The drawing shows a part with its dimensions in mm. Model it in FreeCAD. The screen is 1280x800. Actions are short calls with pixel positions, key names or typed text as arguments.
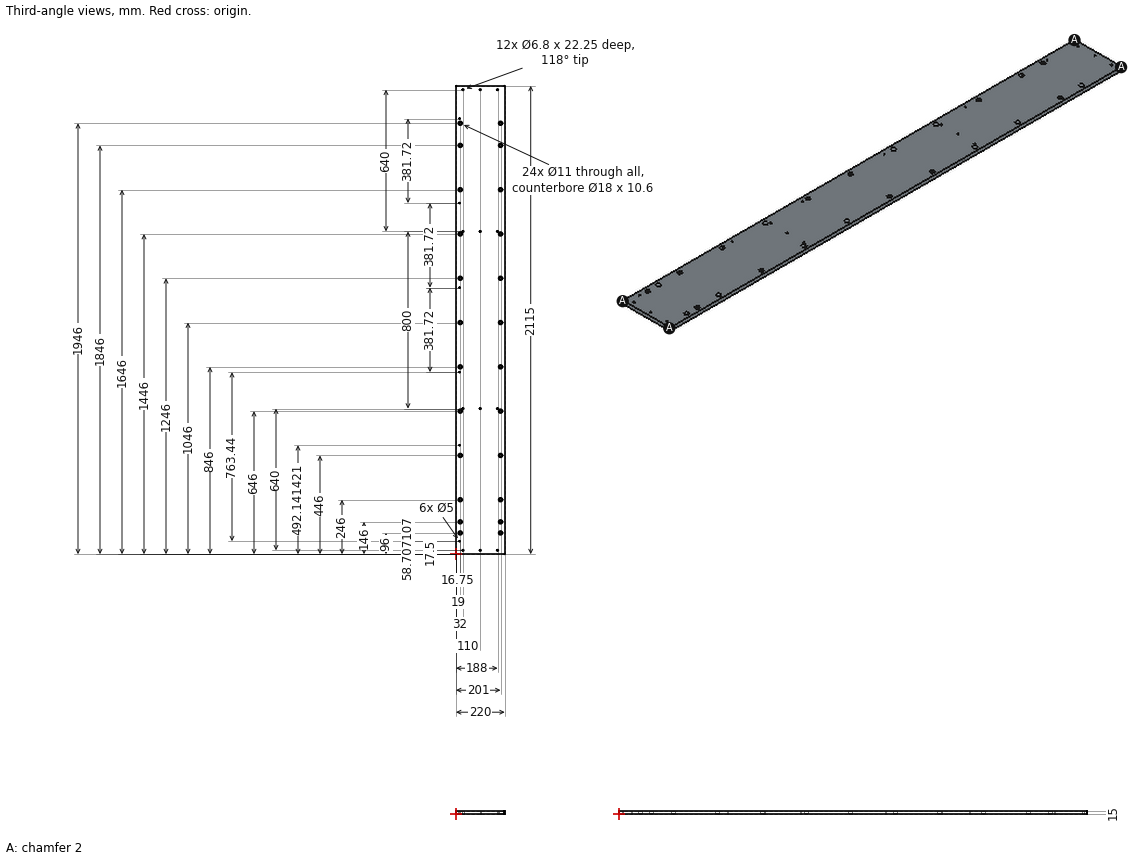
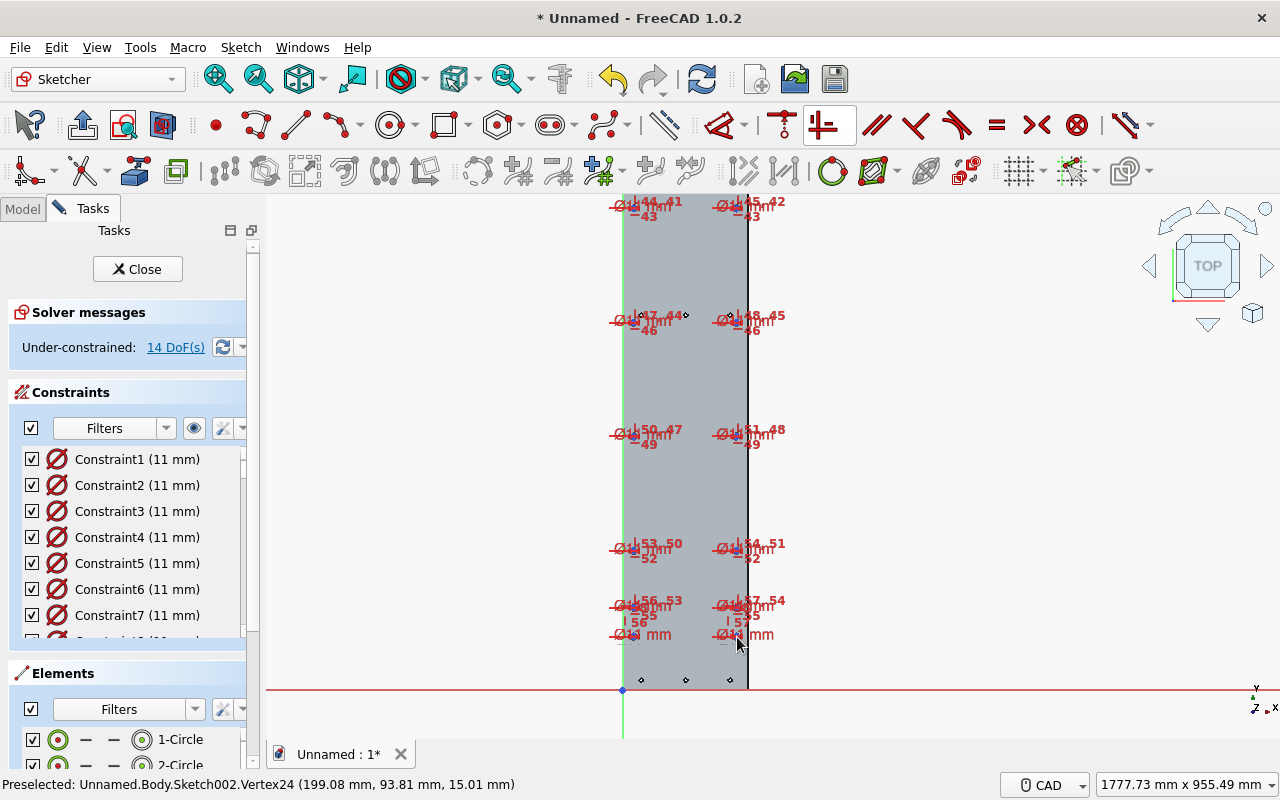
click(720, 126)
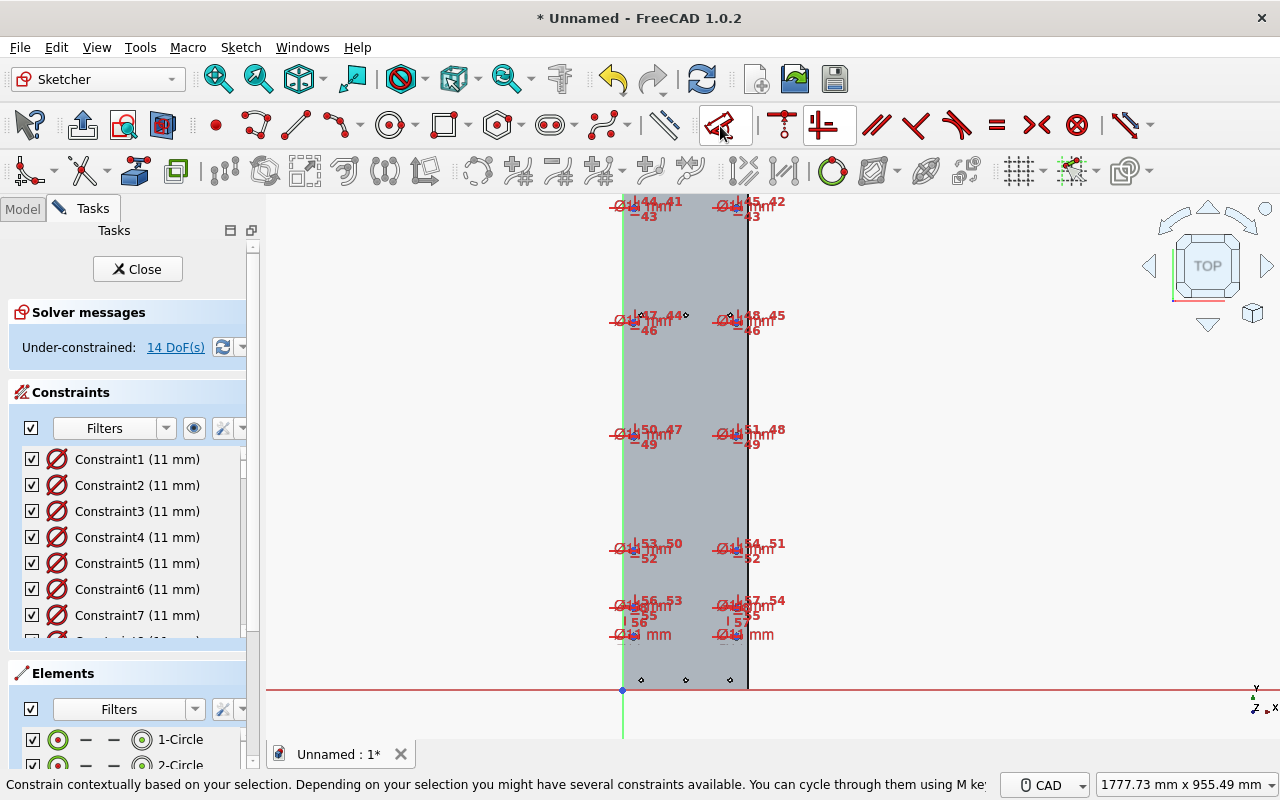
scroll(714, 610, down, 6)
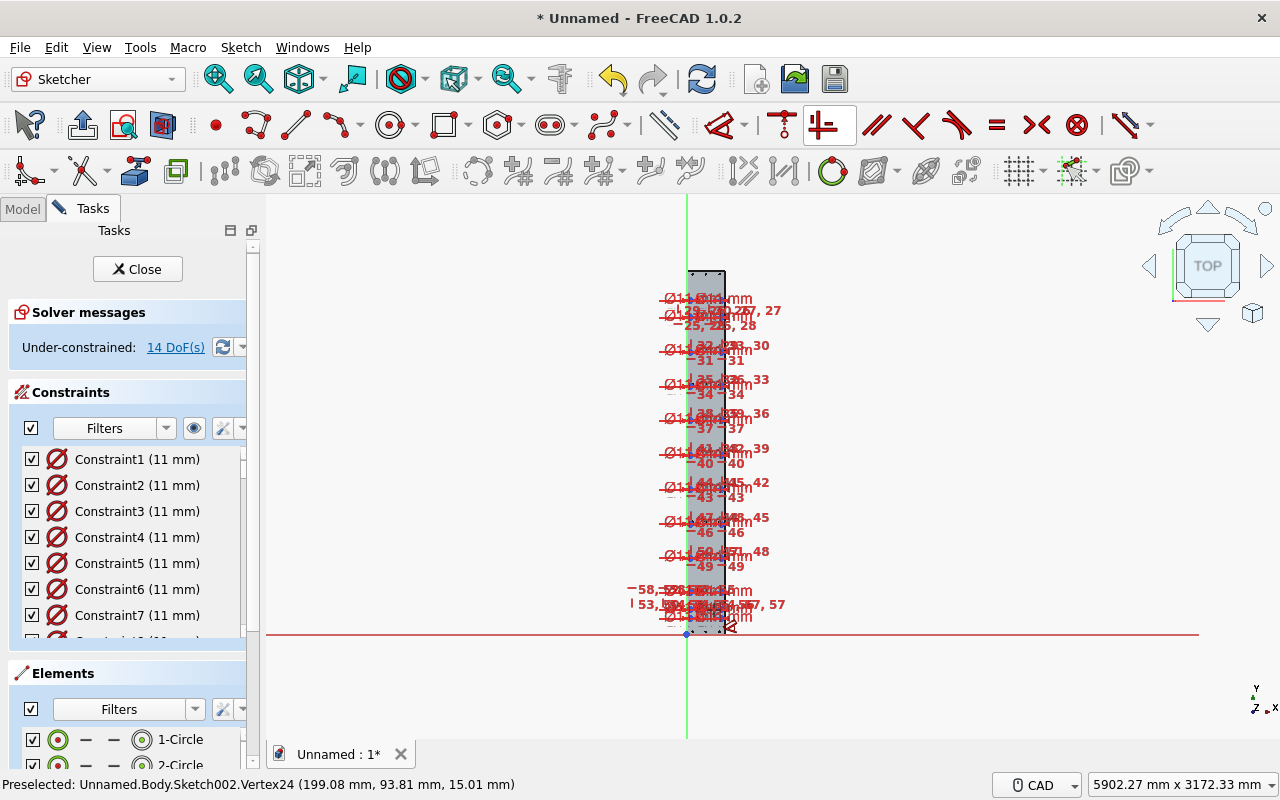
scroll(690, 301, up, 13)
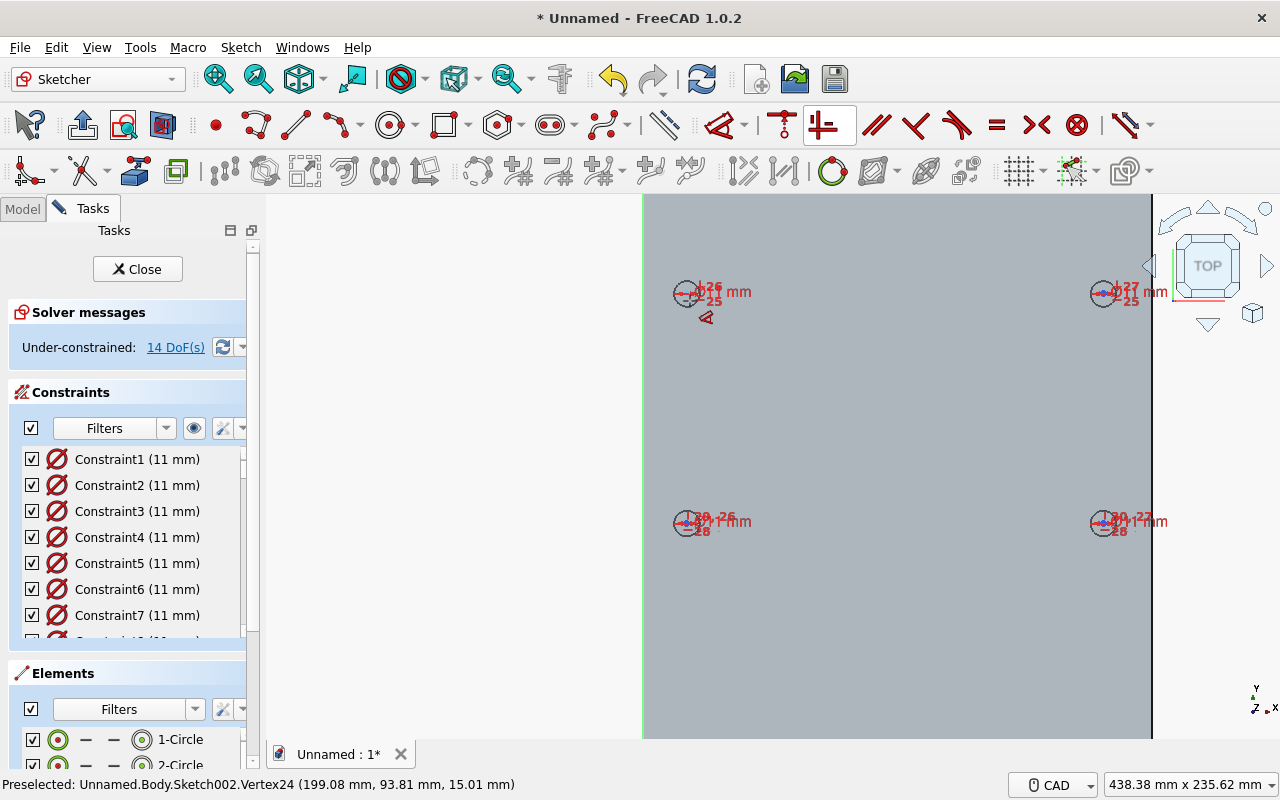
click(687, 294)
click(665, 260)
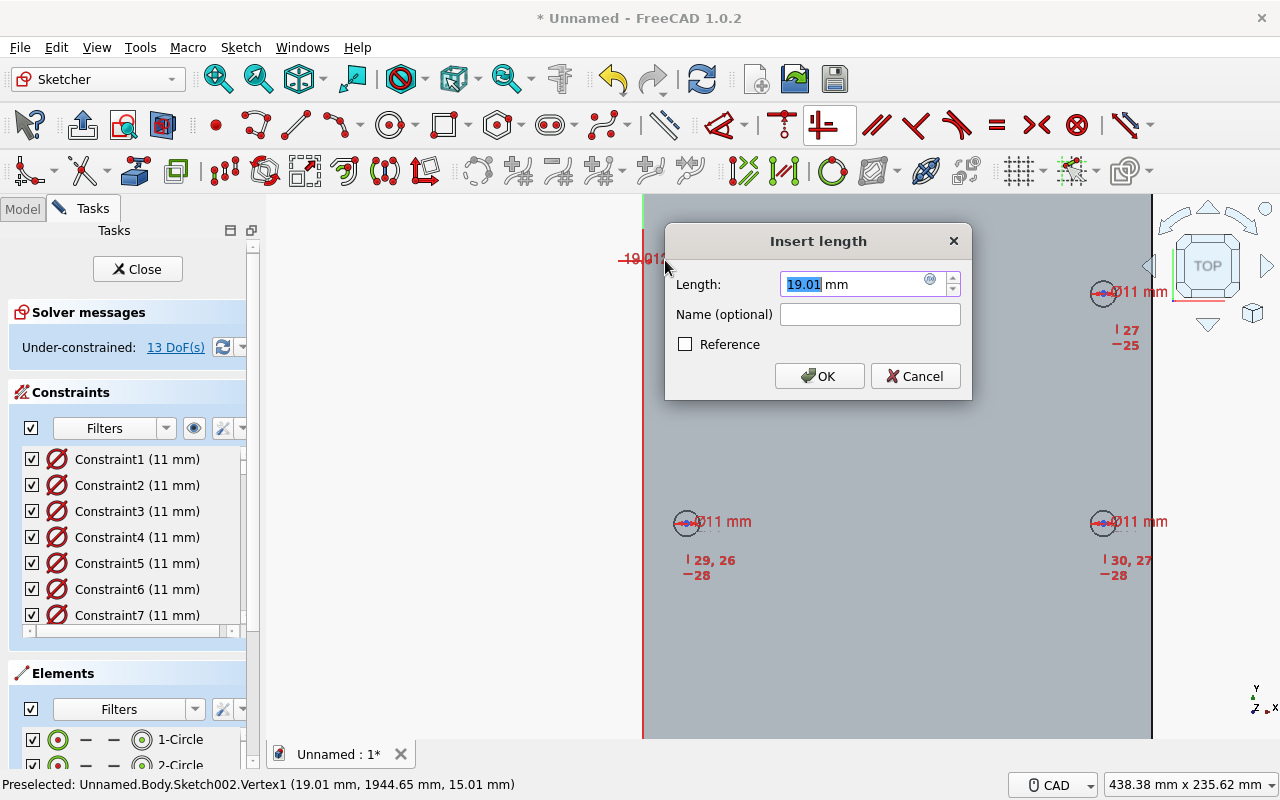
text(19)
key(Return)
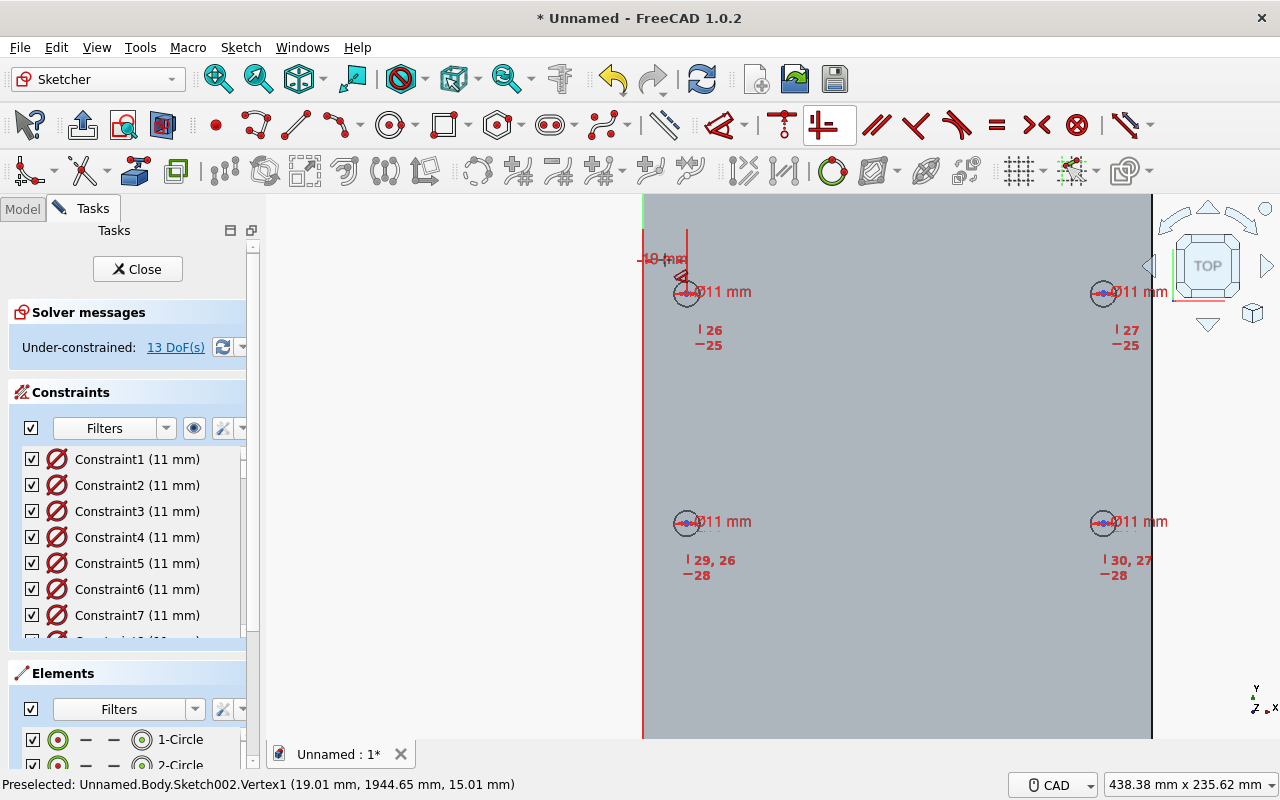
scroll(690, 301, down, 13)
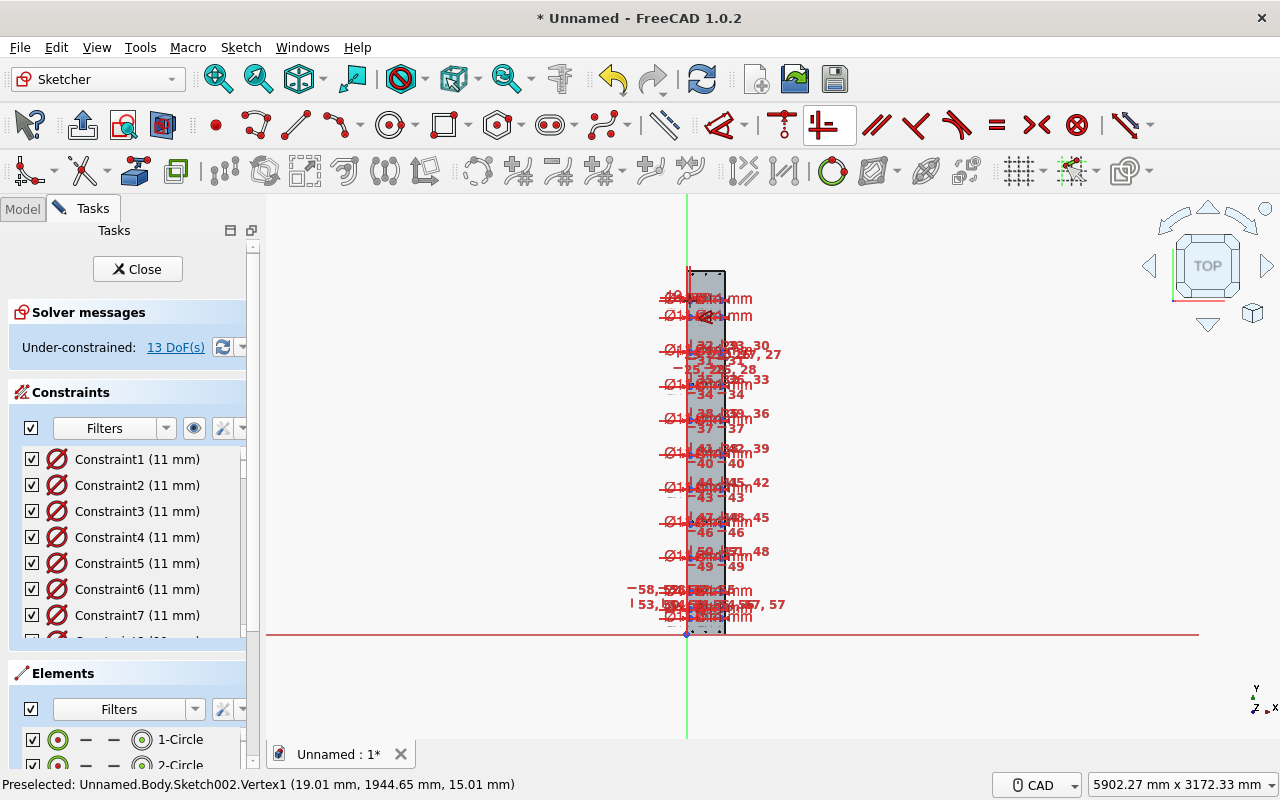
scroll(690, 619, up, 5)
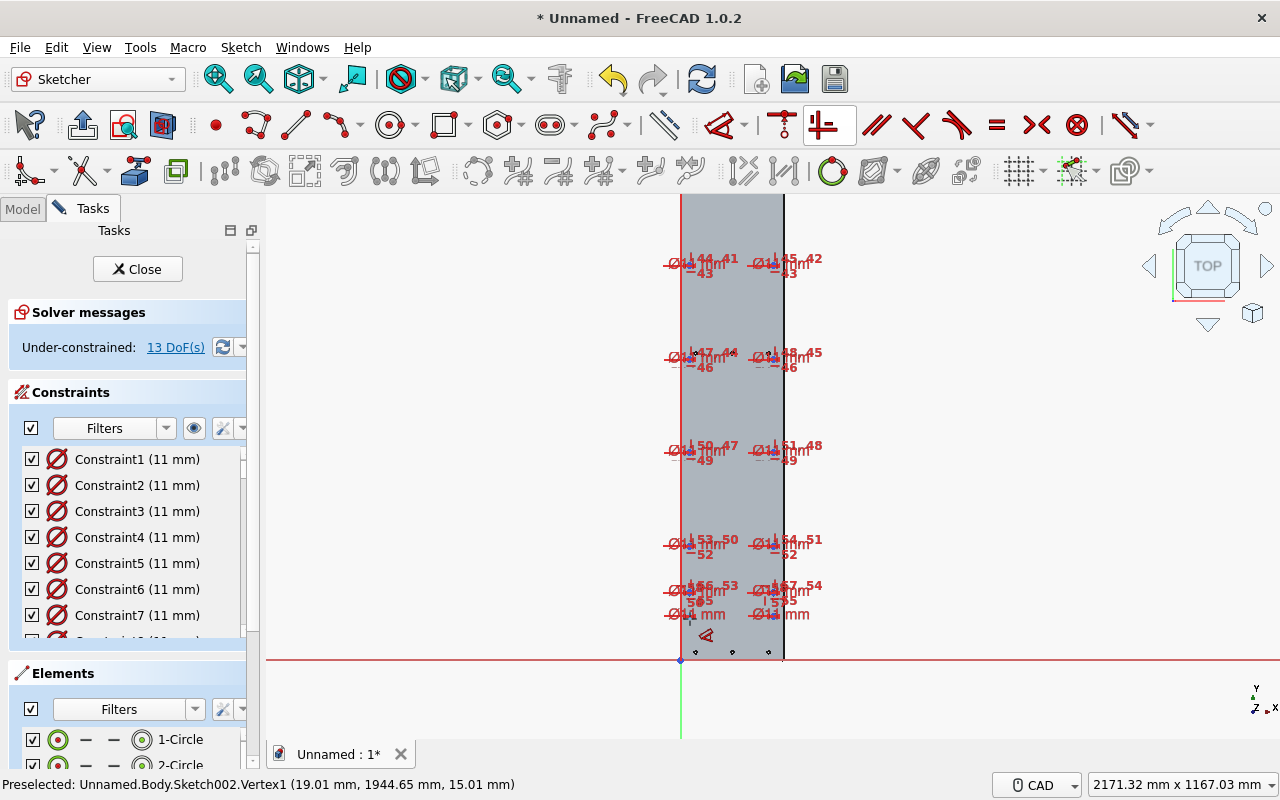
click(690, 616)
click(647, 638)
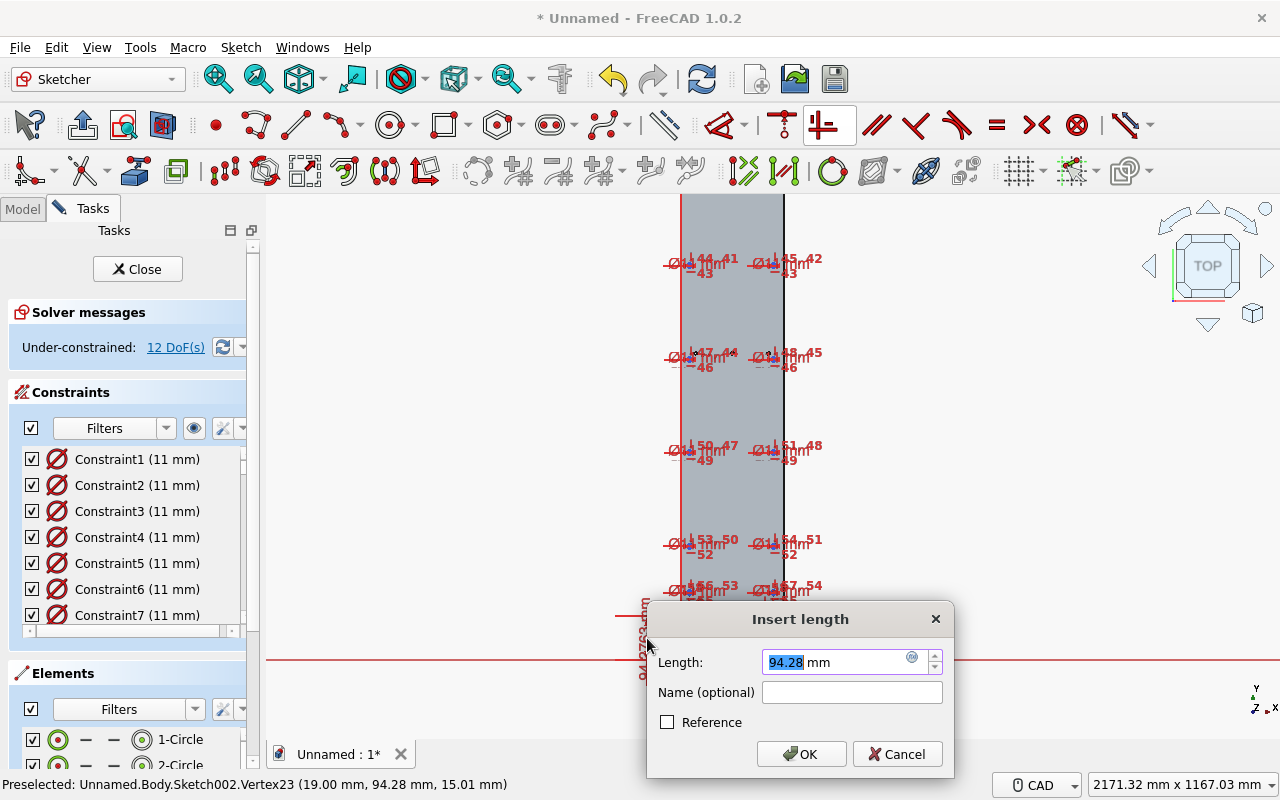
text(96)
key(Return)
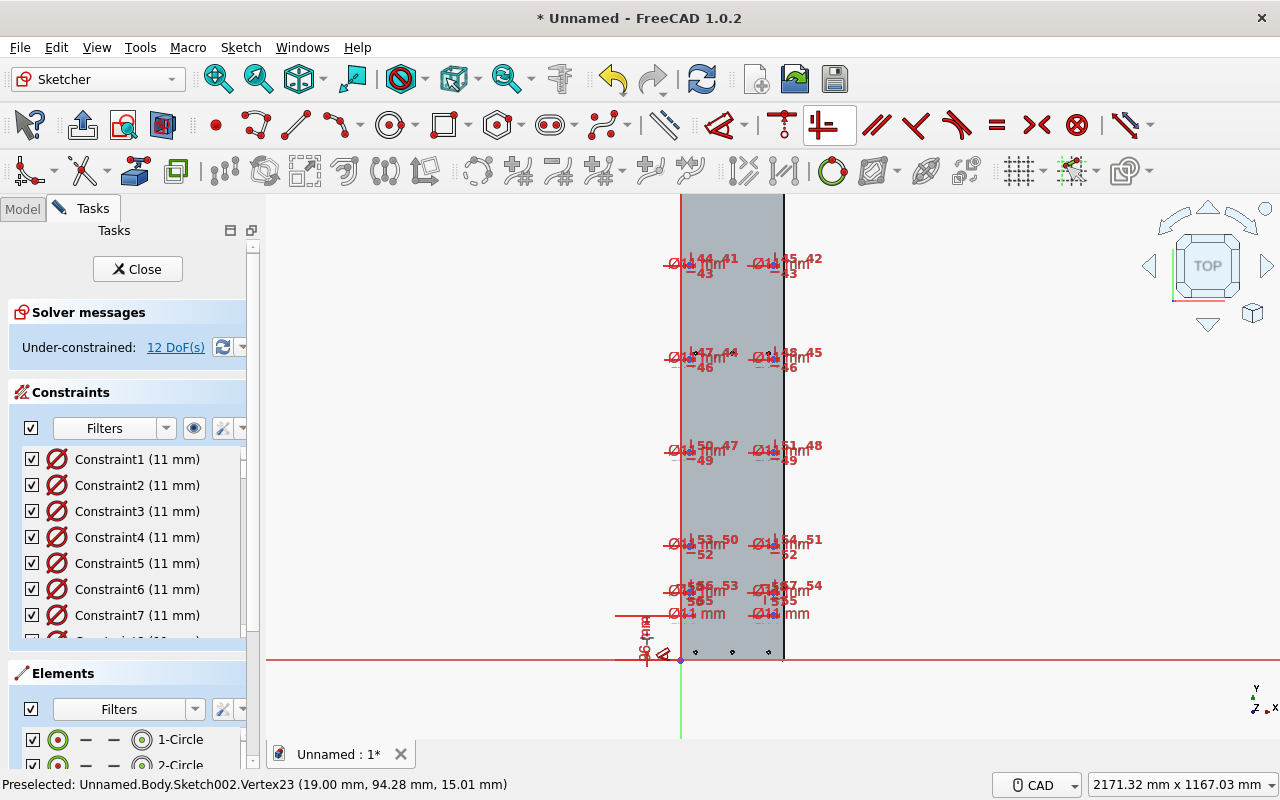
scroll(690, 619, down, 5)